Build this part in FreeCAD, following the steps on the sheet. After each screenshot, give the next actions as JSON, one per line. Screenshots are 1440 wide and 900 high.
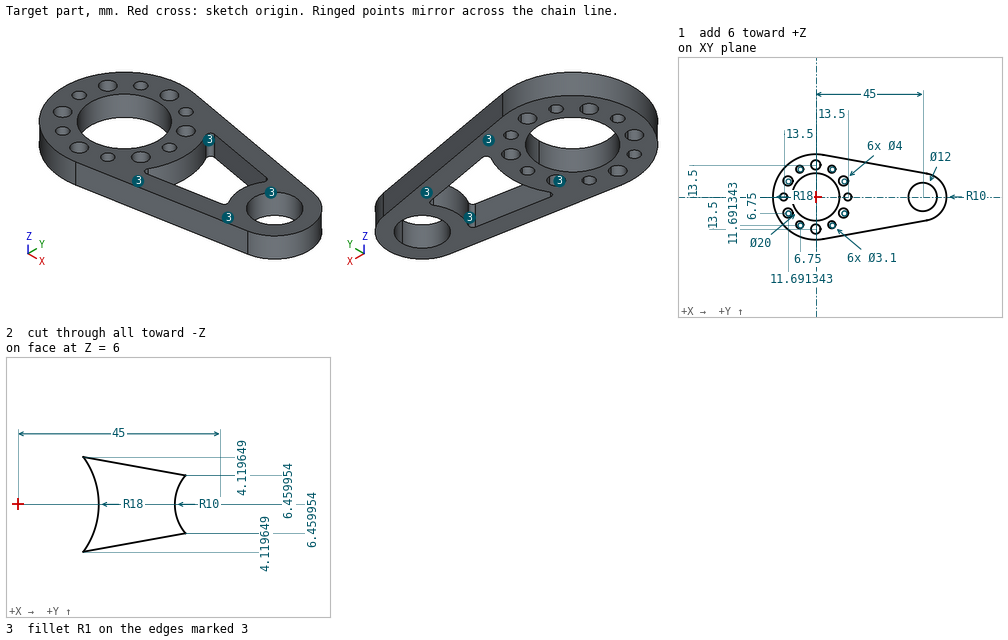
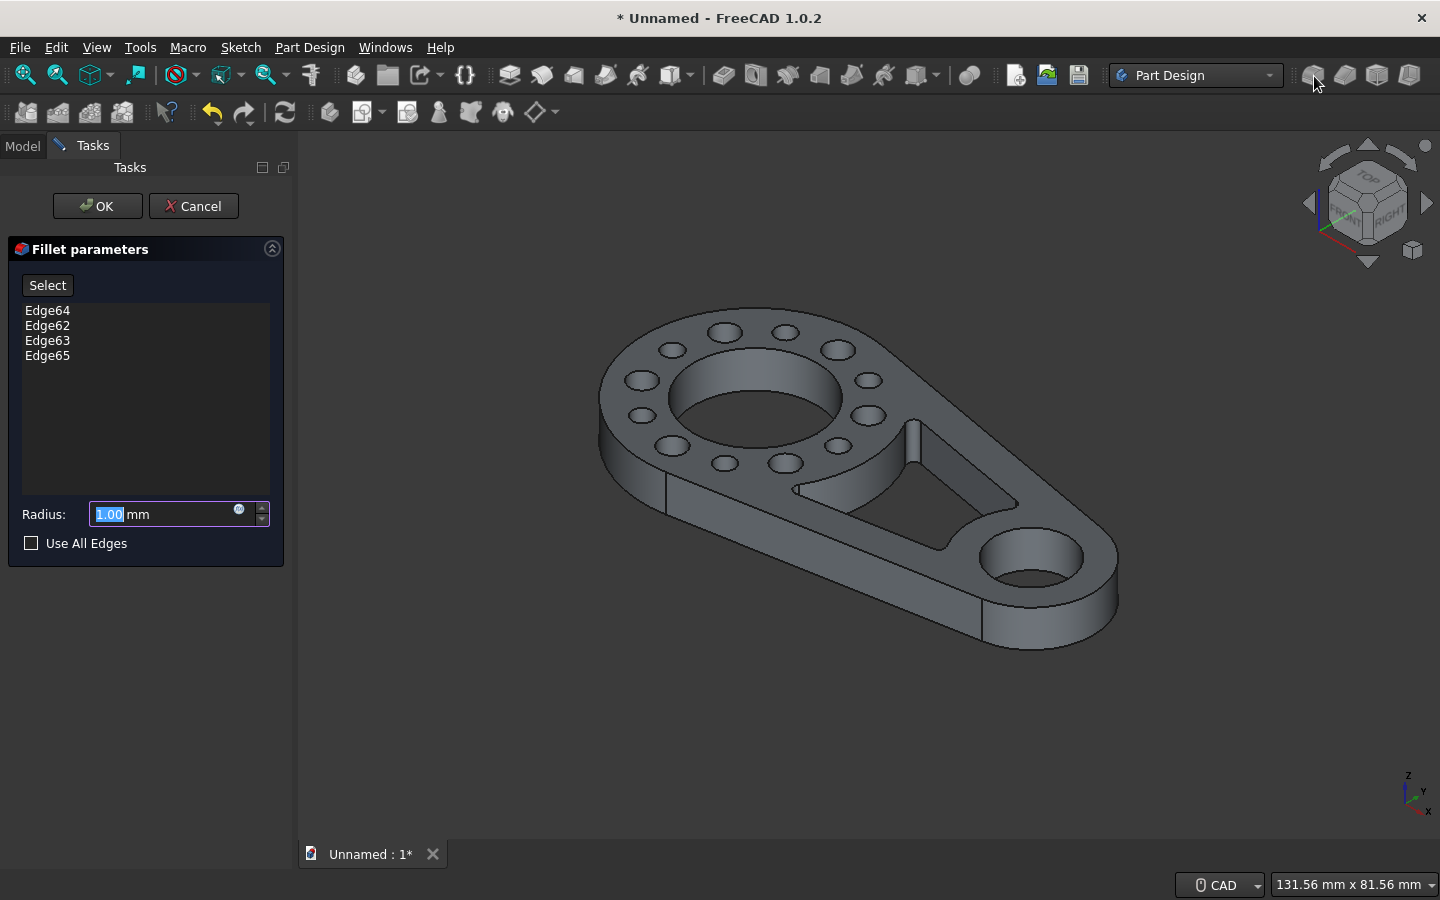
{"action": "type", "text": "1"}
{"action": "key", "text": "Tab"}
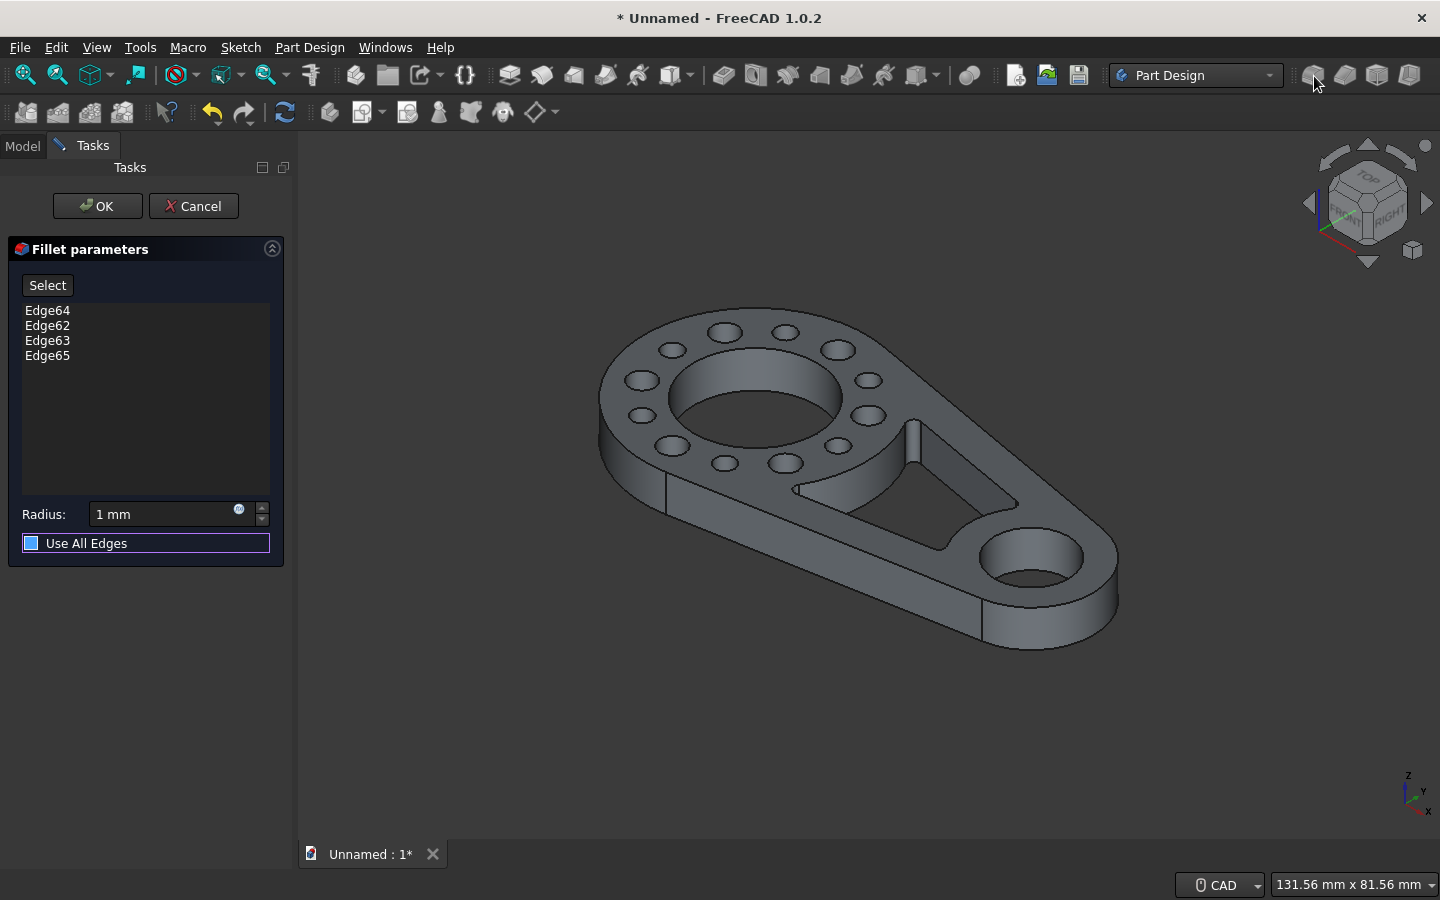
{"action": "left_click", "coordinate": [98, 206]}